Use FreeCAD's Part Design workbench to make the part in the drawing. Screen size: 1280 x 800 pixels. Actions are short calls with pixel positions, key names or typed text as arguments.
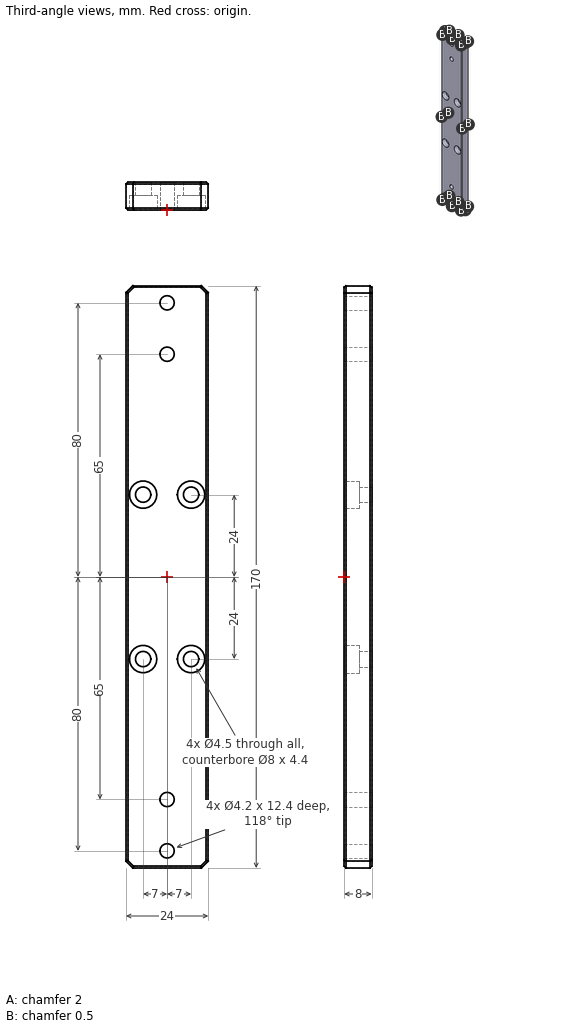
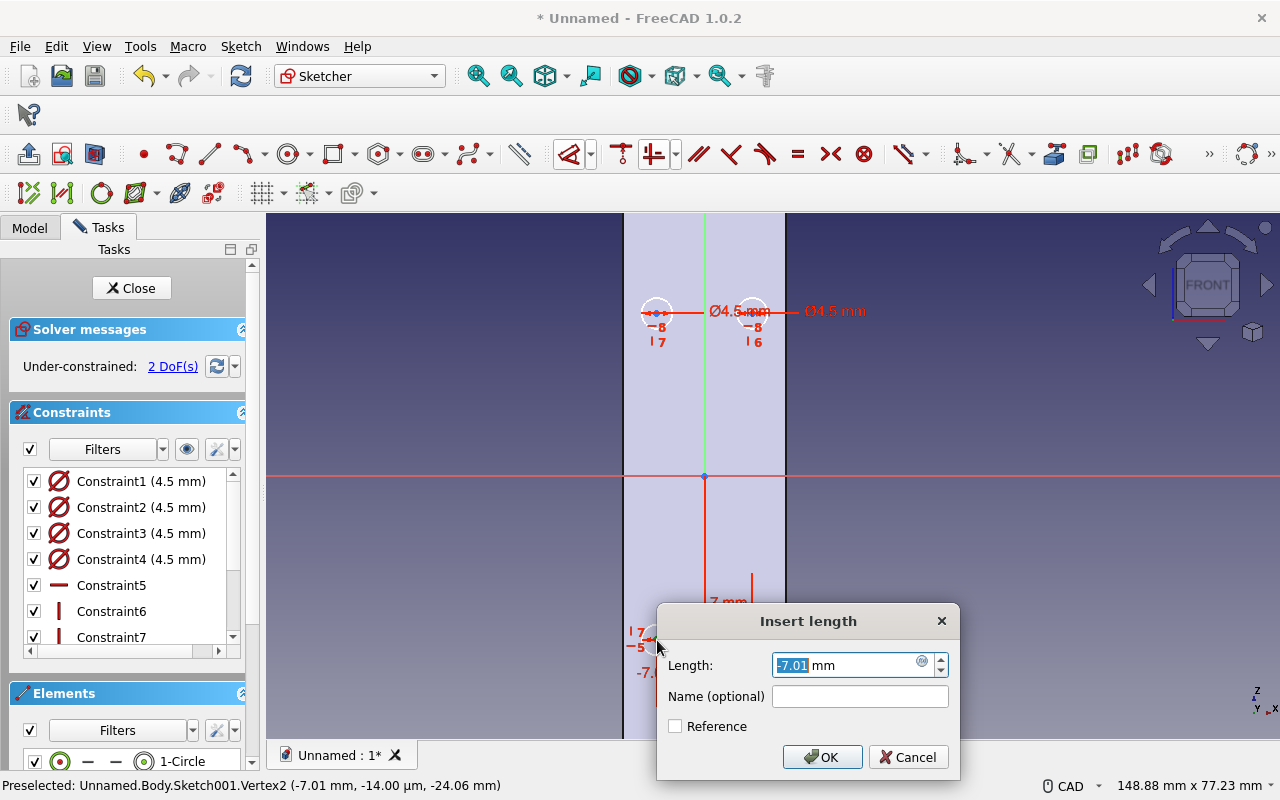
text(-7)
key(Return)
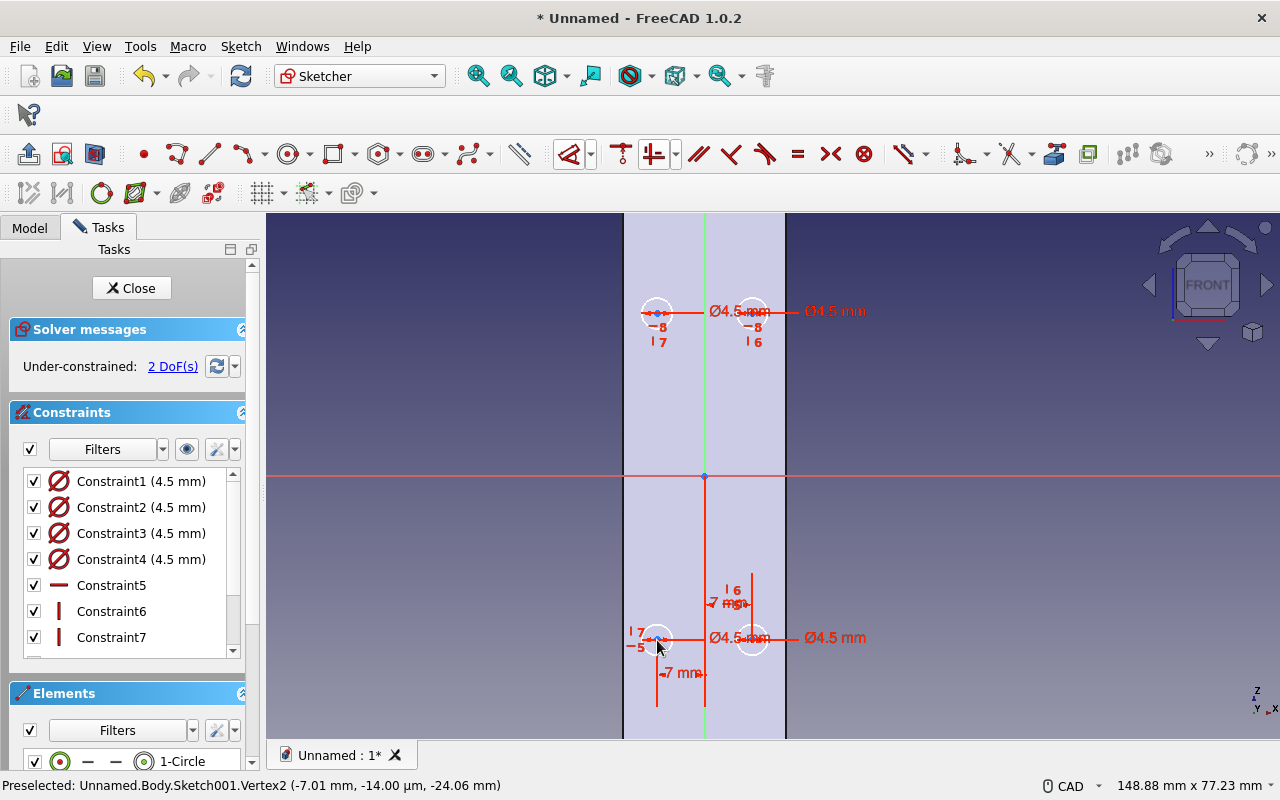
click(752, 640)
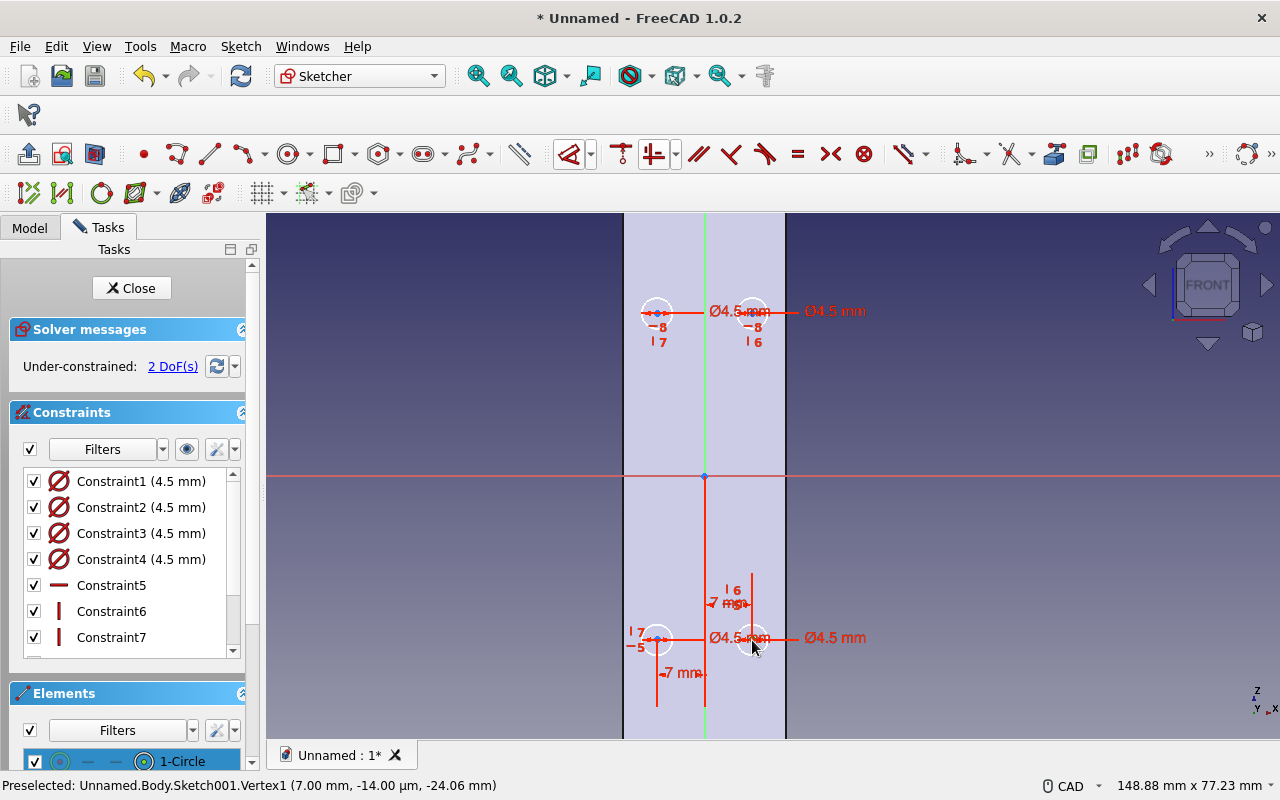
click(590, 154)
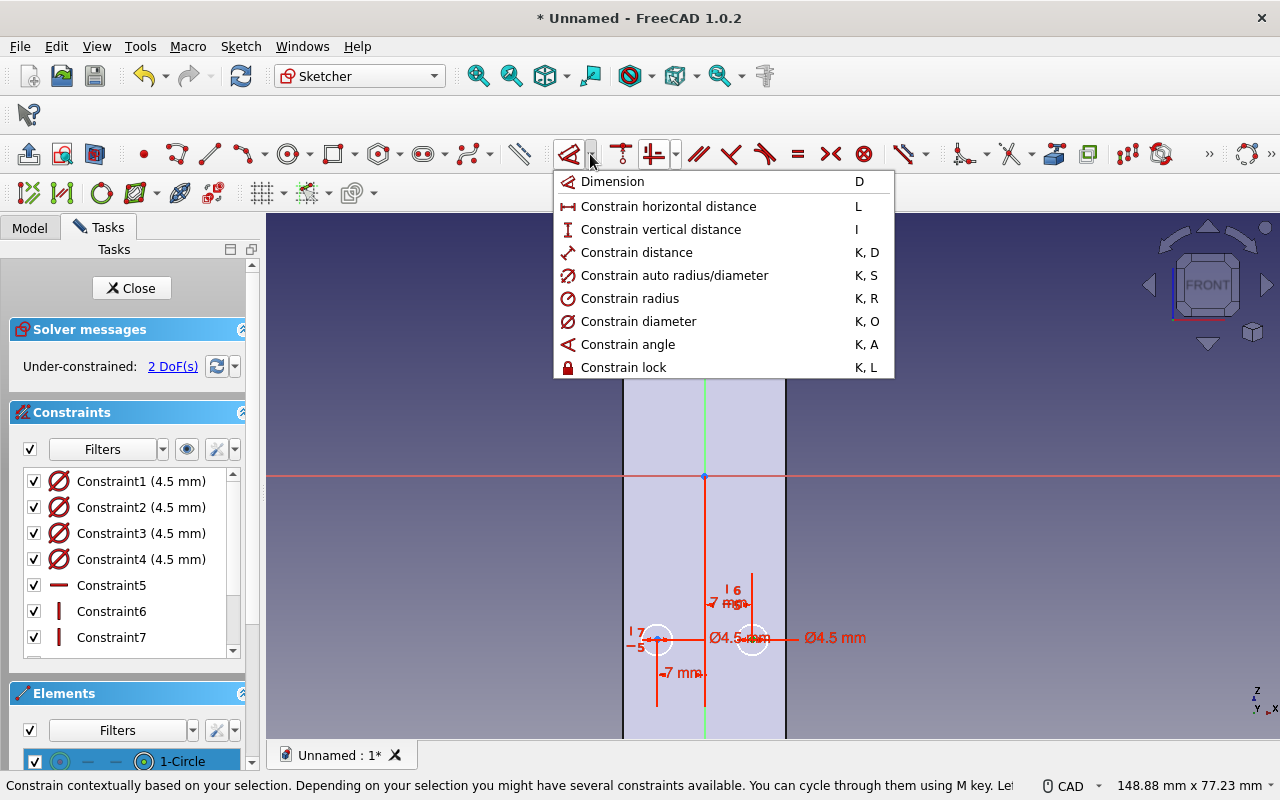
click(724, 230)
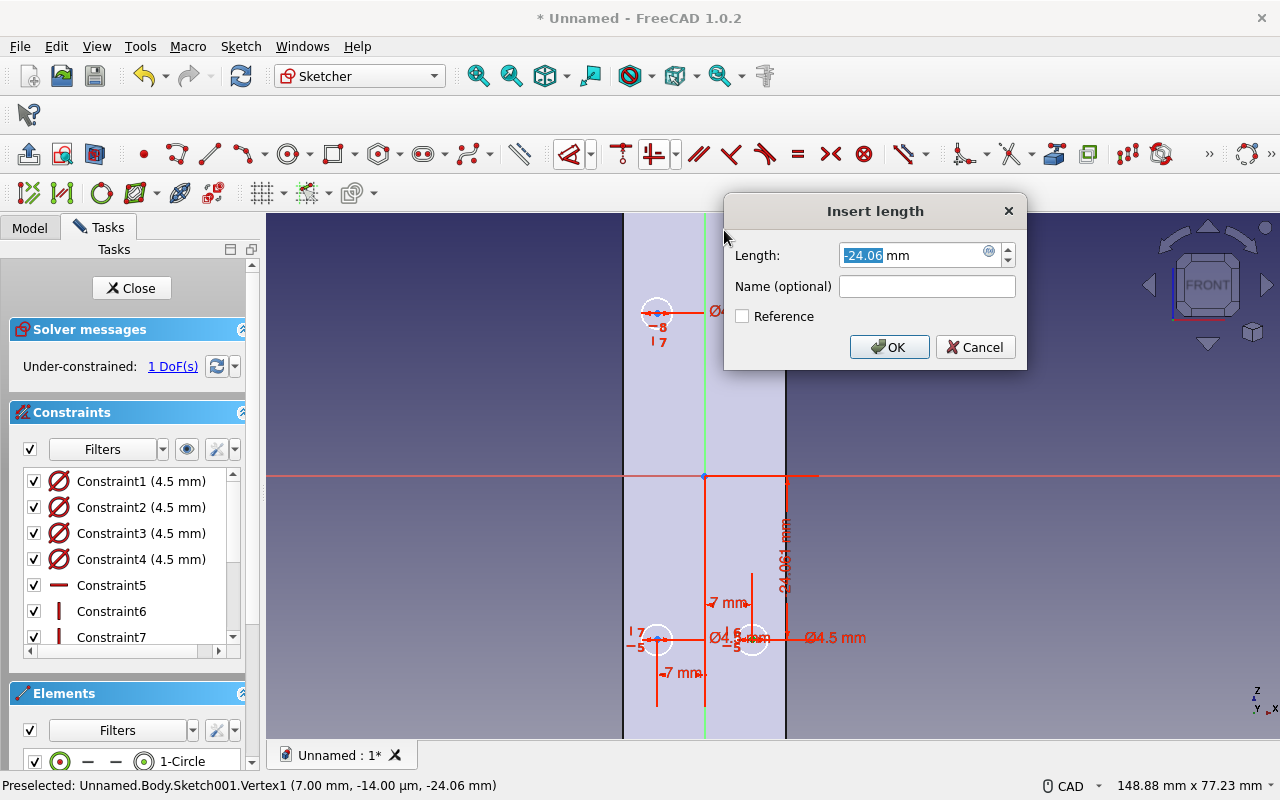
text(-24)
key(Return)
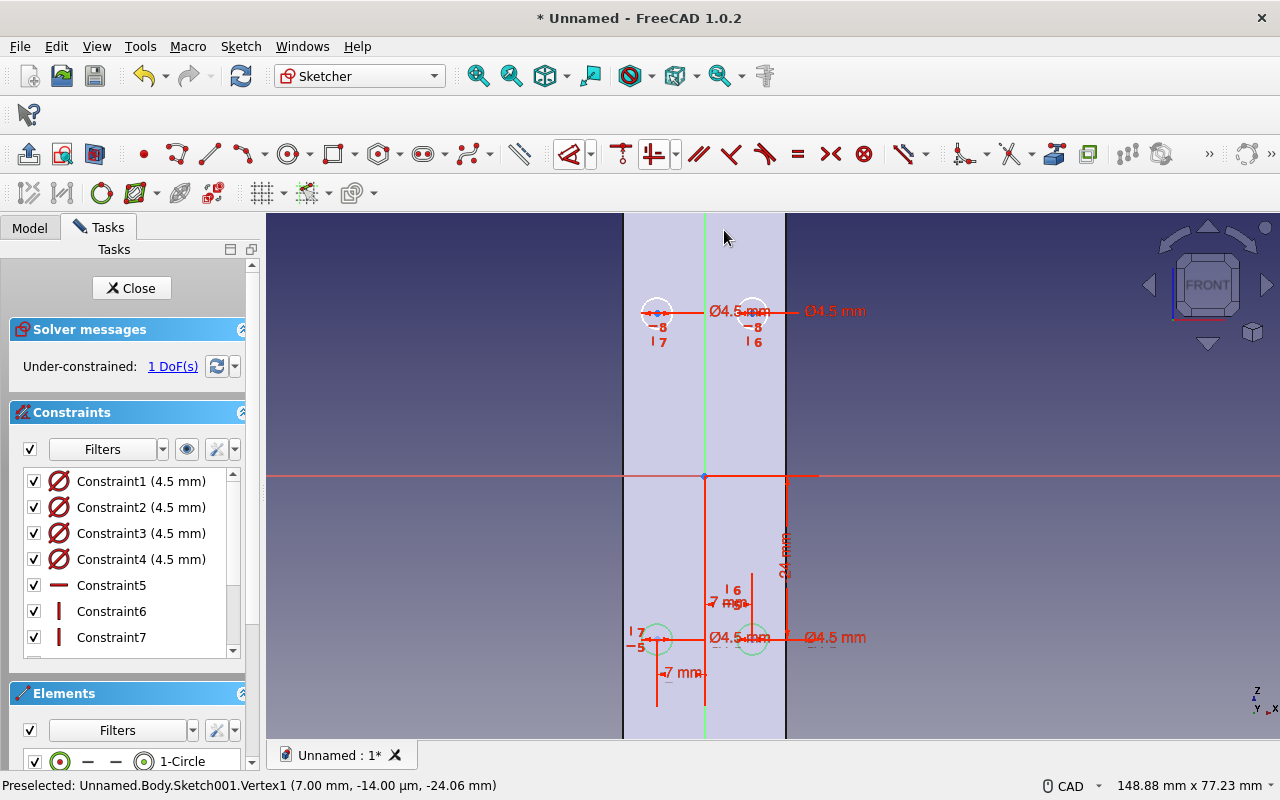
click(752, 313)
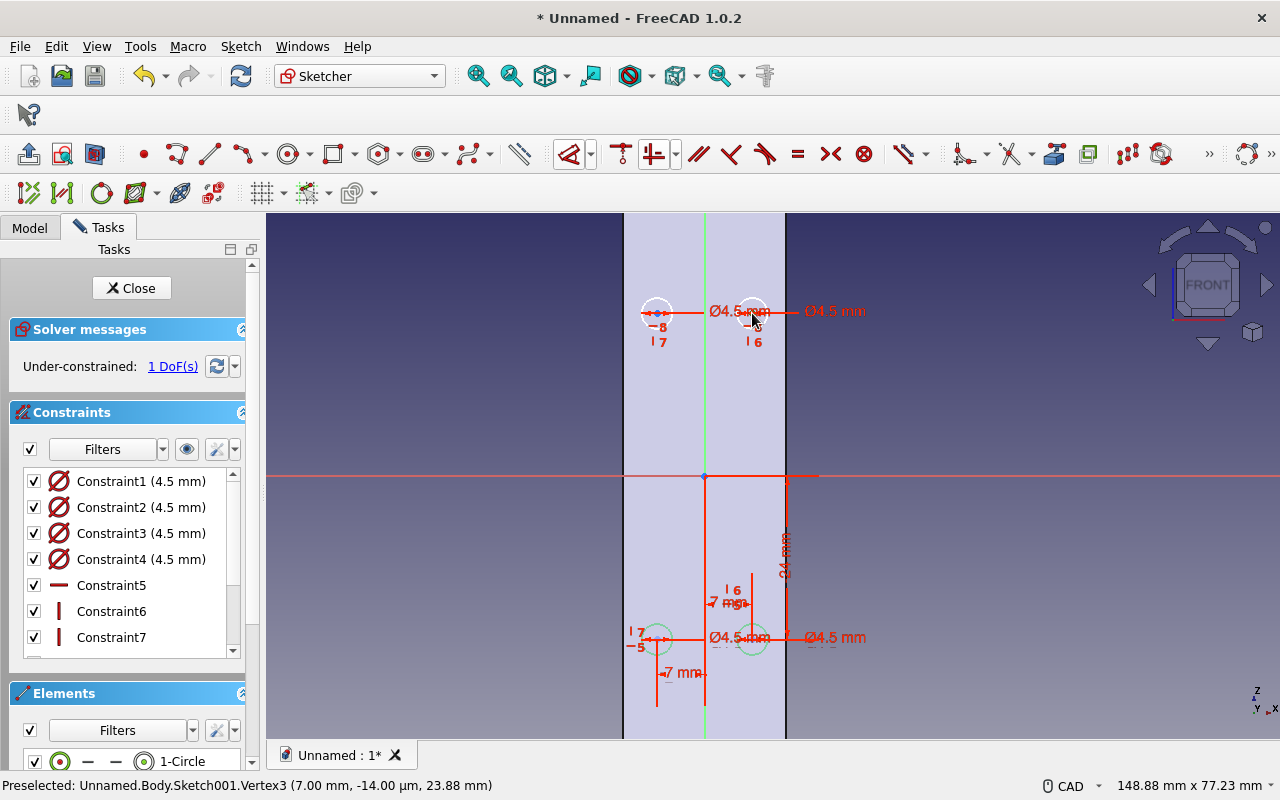
key(i)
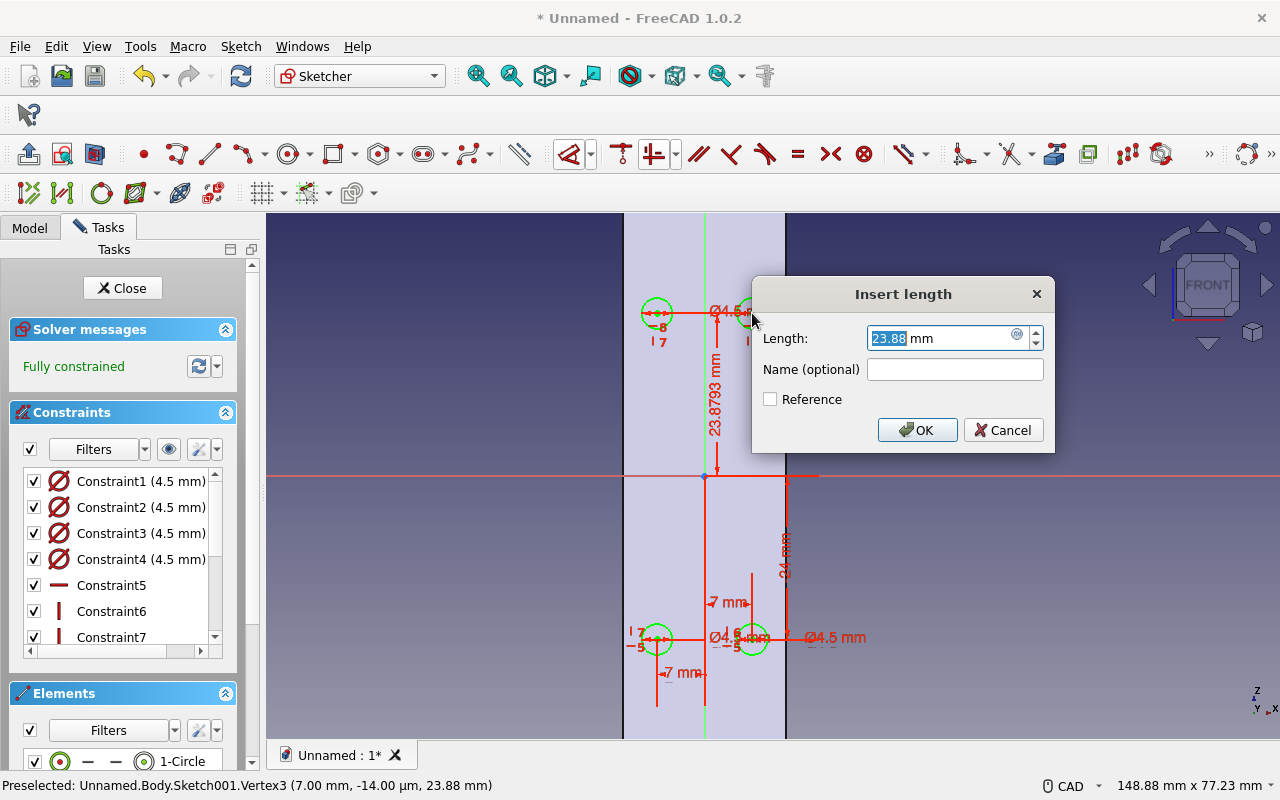
text(24)
key(Return)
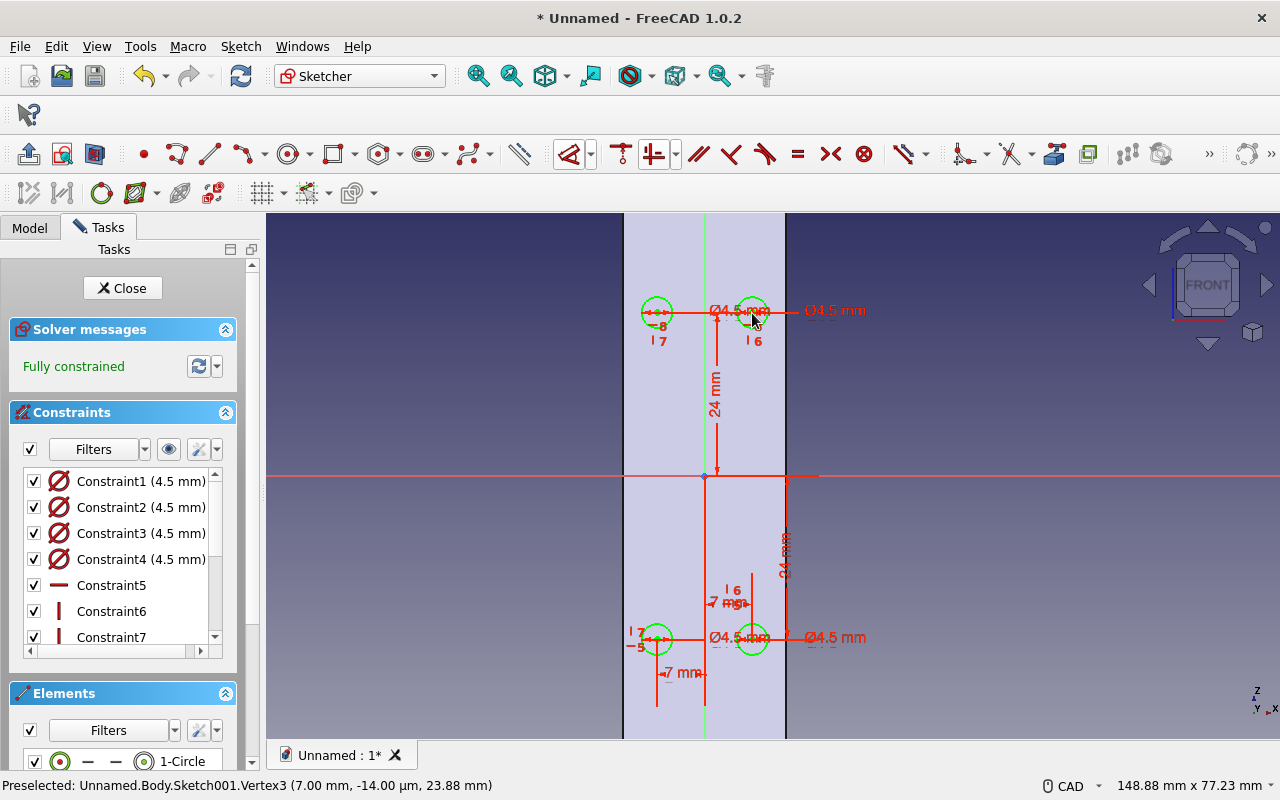
click(123, 288)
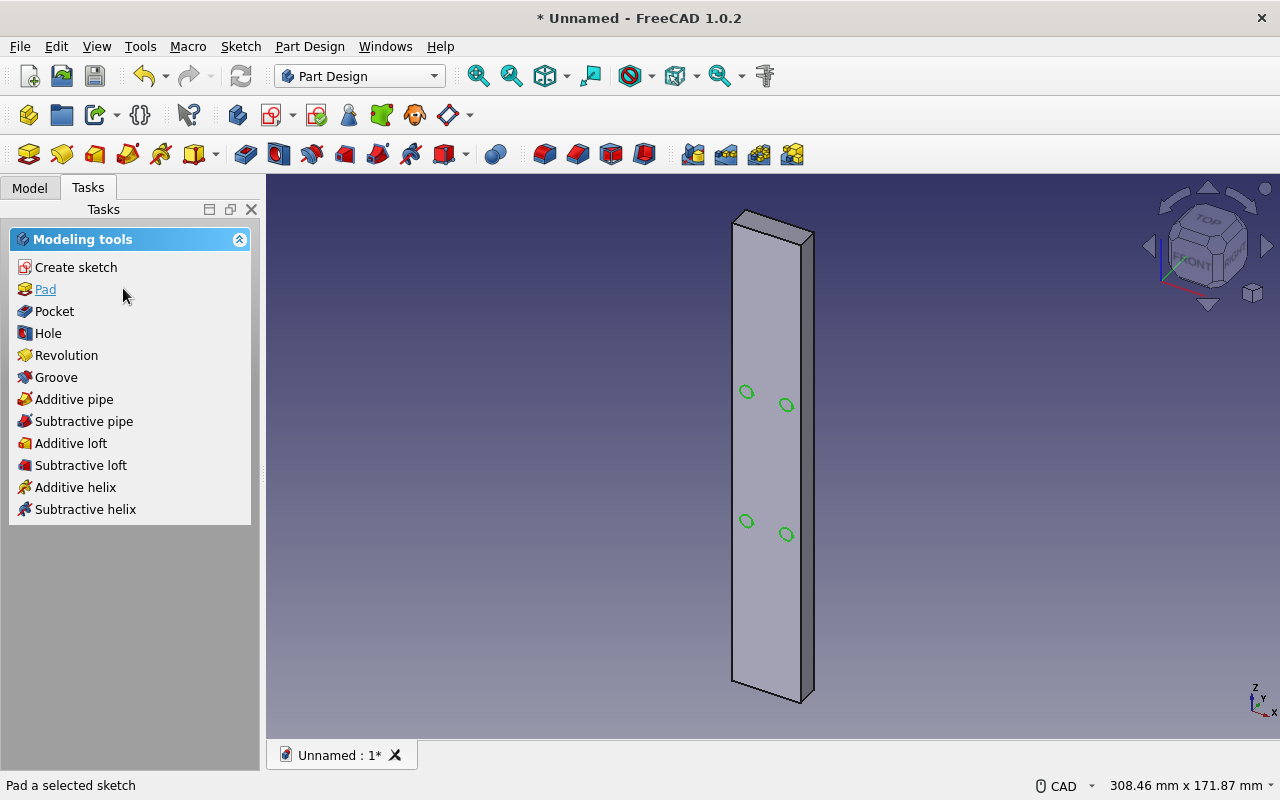
click(279, 154)